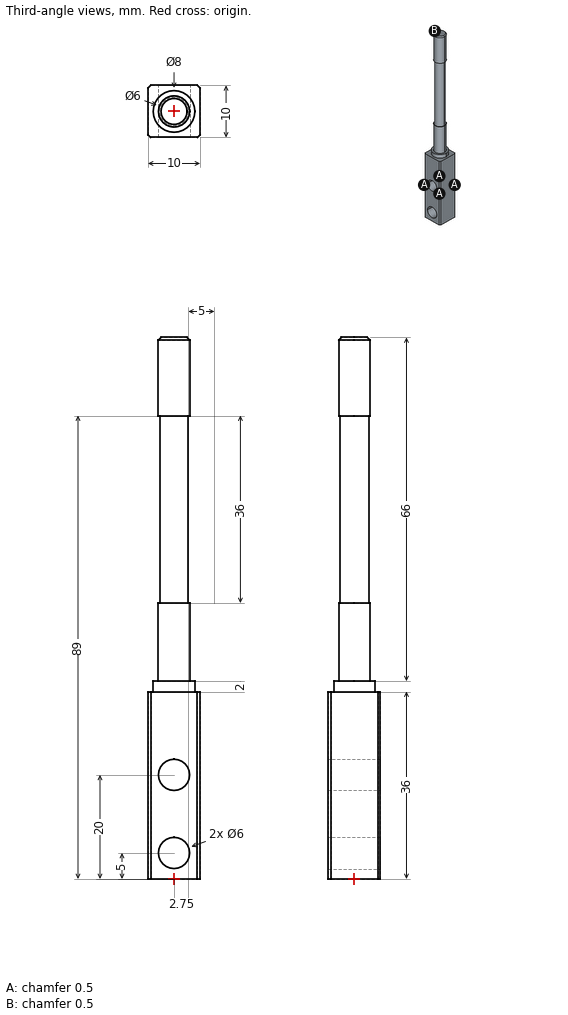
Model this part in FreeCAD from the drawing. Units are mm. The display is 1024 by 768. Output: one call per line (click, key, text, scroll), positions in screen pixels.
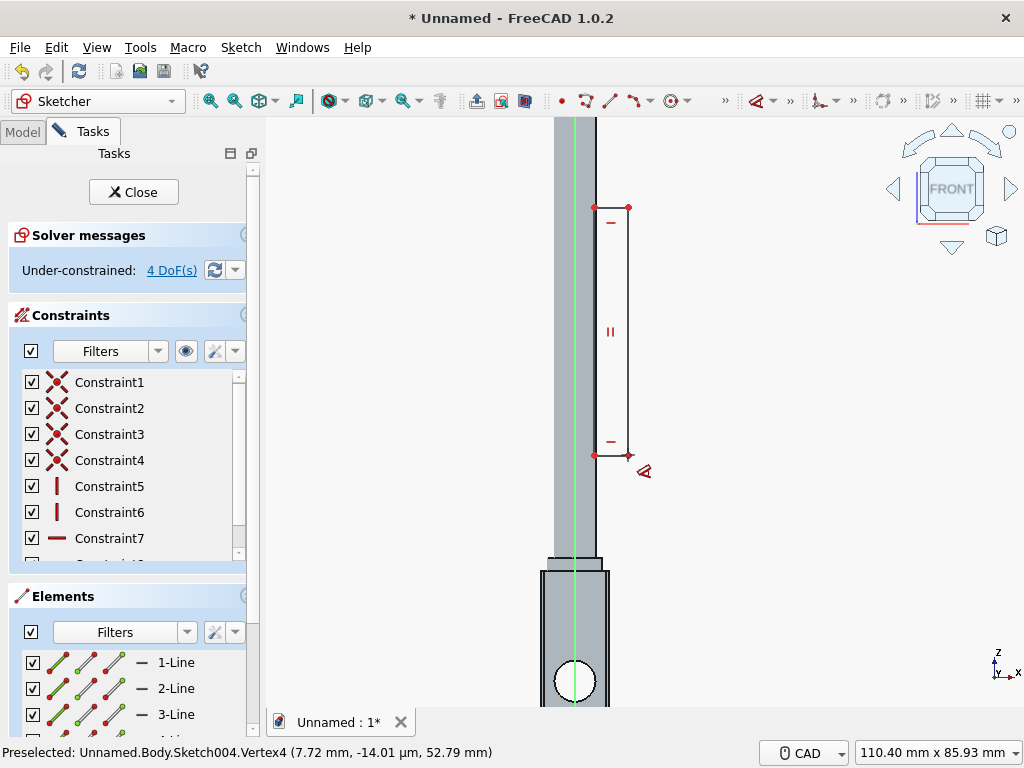
scroll(604, 456, up, 2)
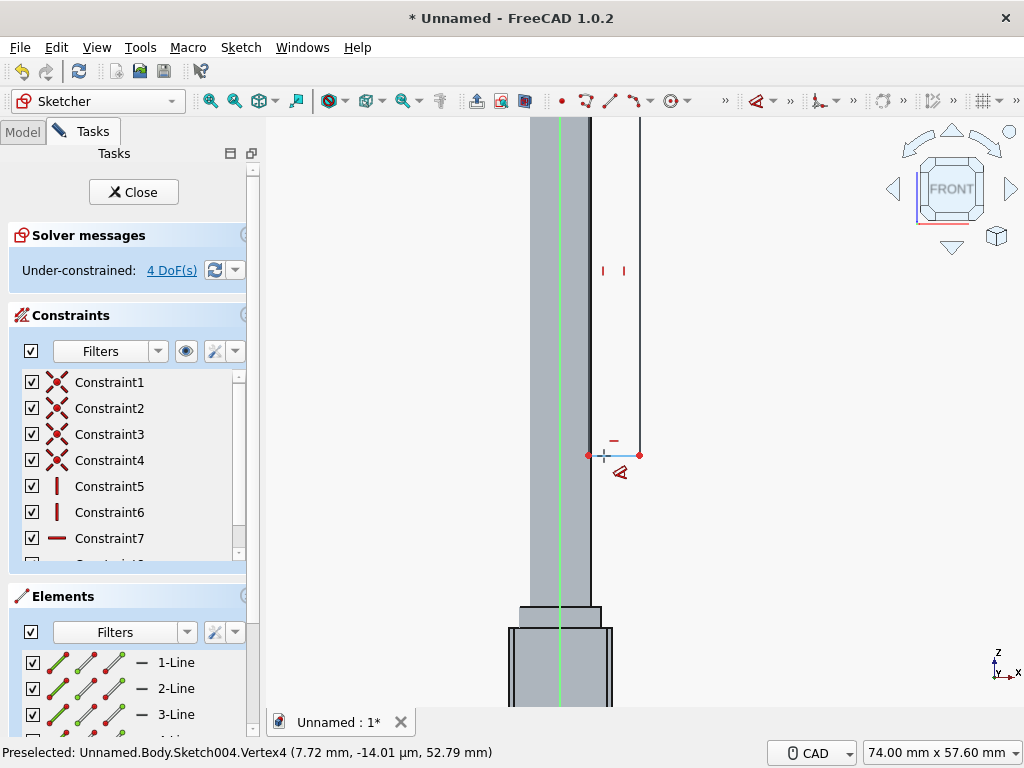
click(604, 456)
click(614, 422)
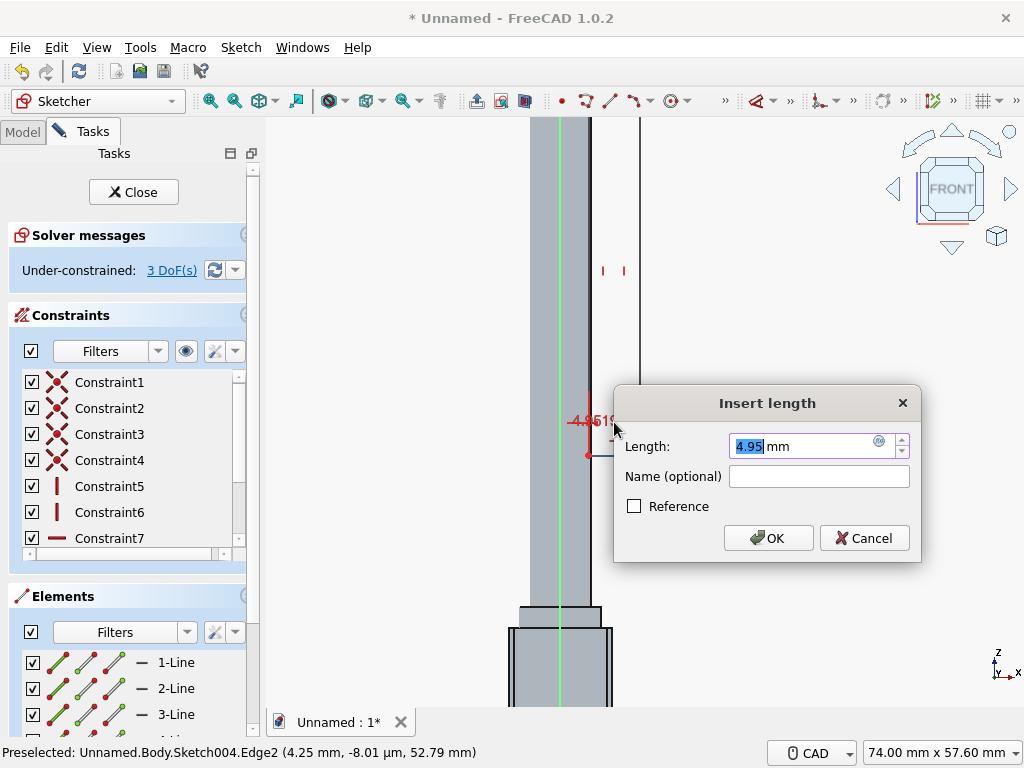
text(5)
key(Return)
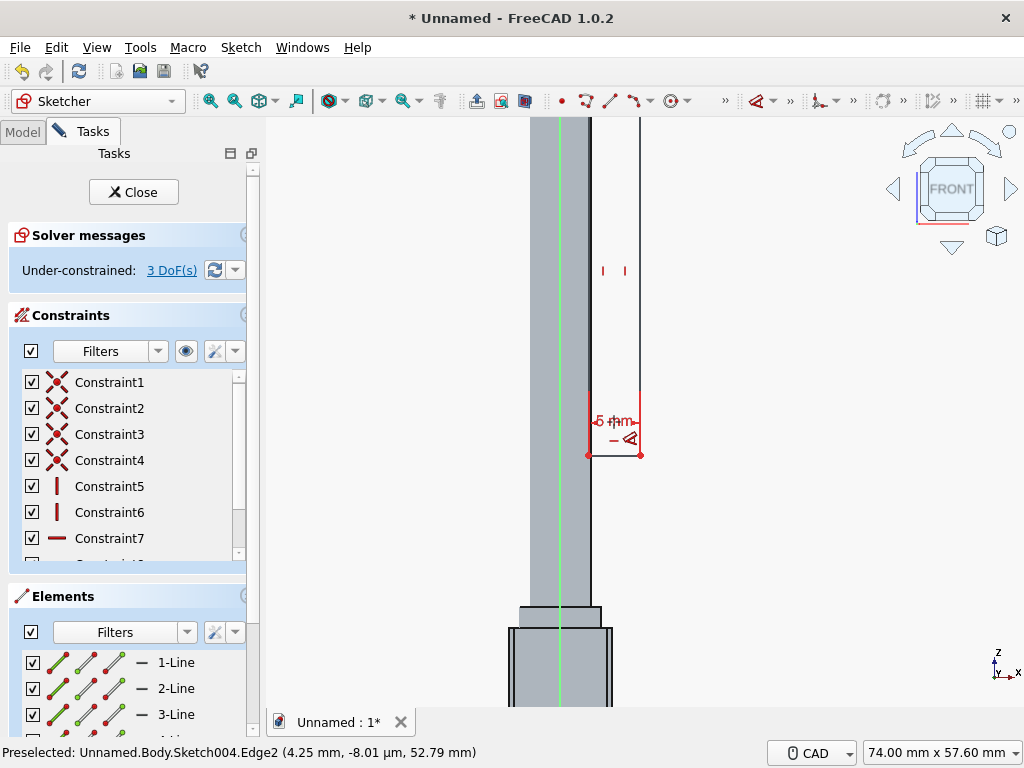
click(589, 197)
click(623, 300)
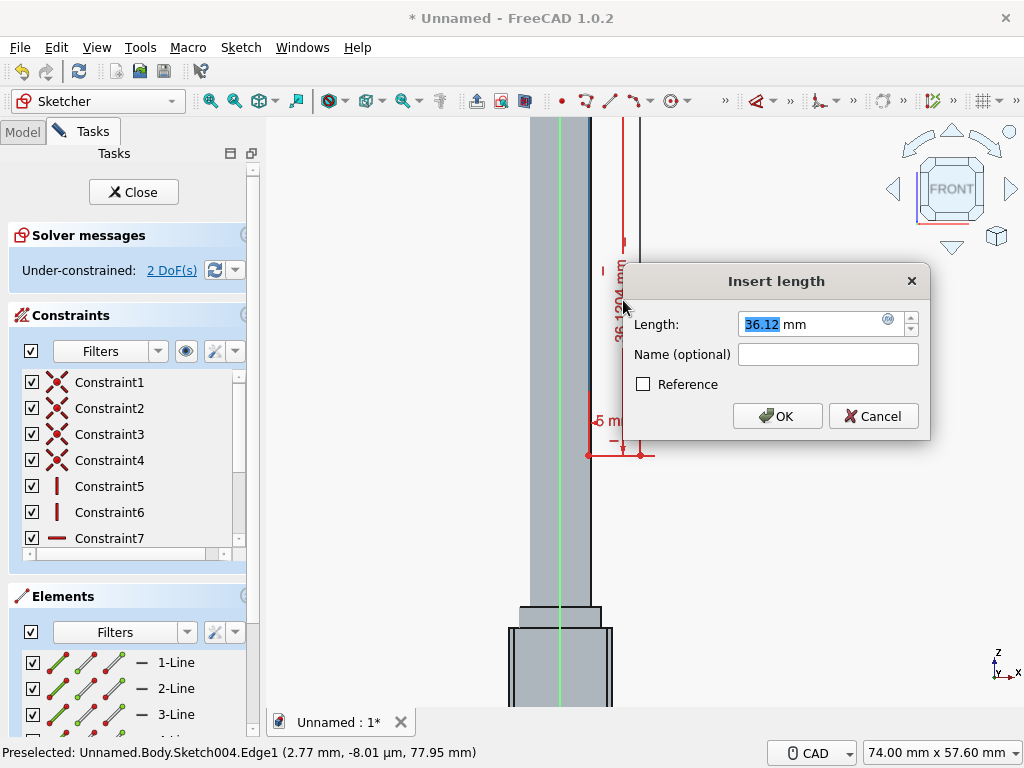
text(36)
key(Return)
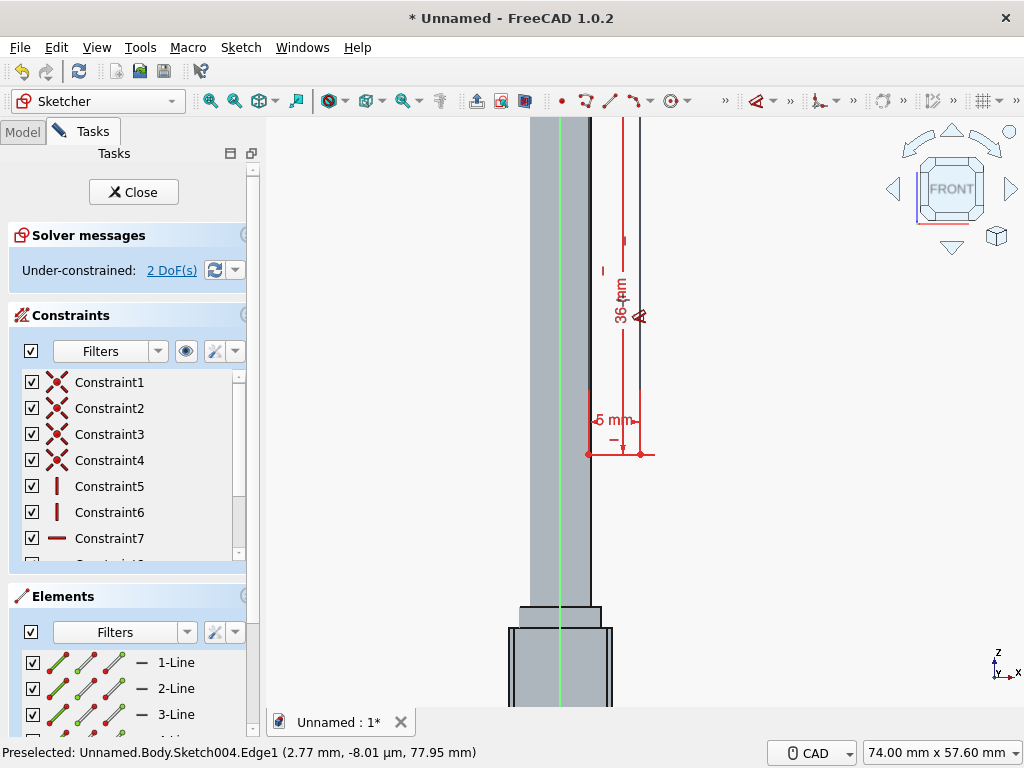
scroll(557, 307, down, 4)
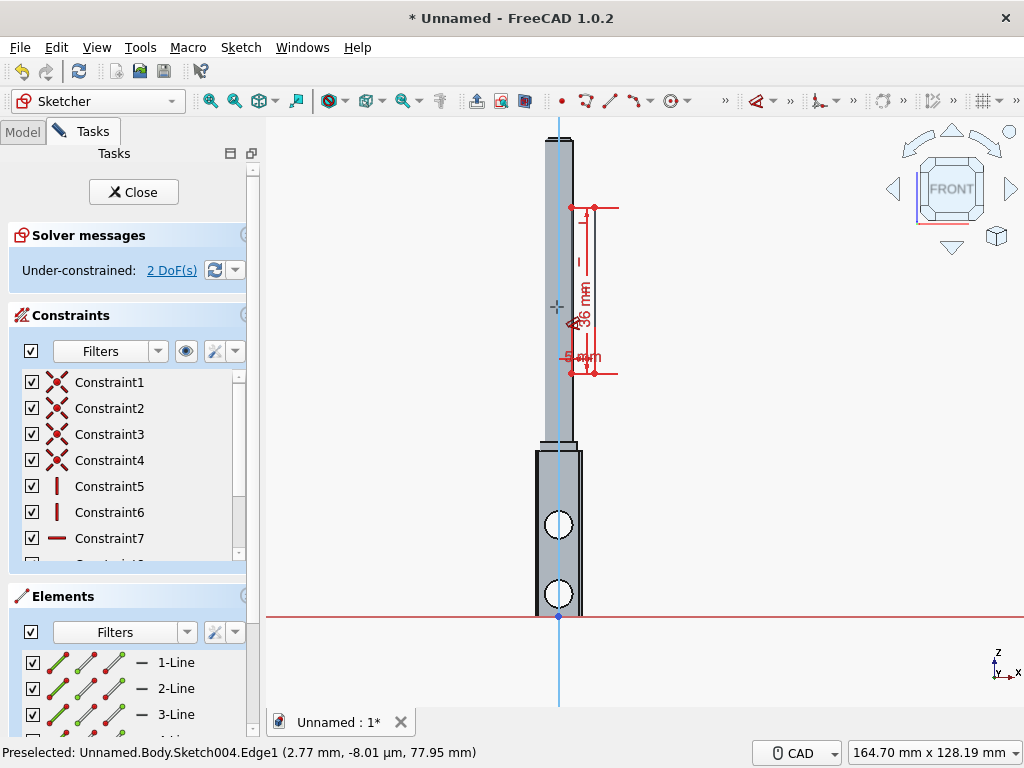
click(572, 208)
click(525, 412)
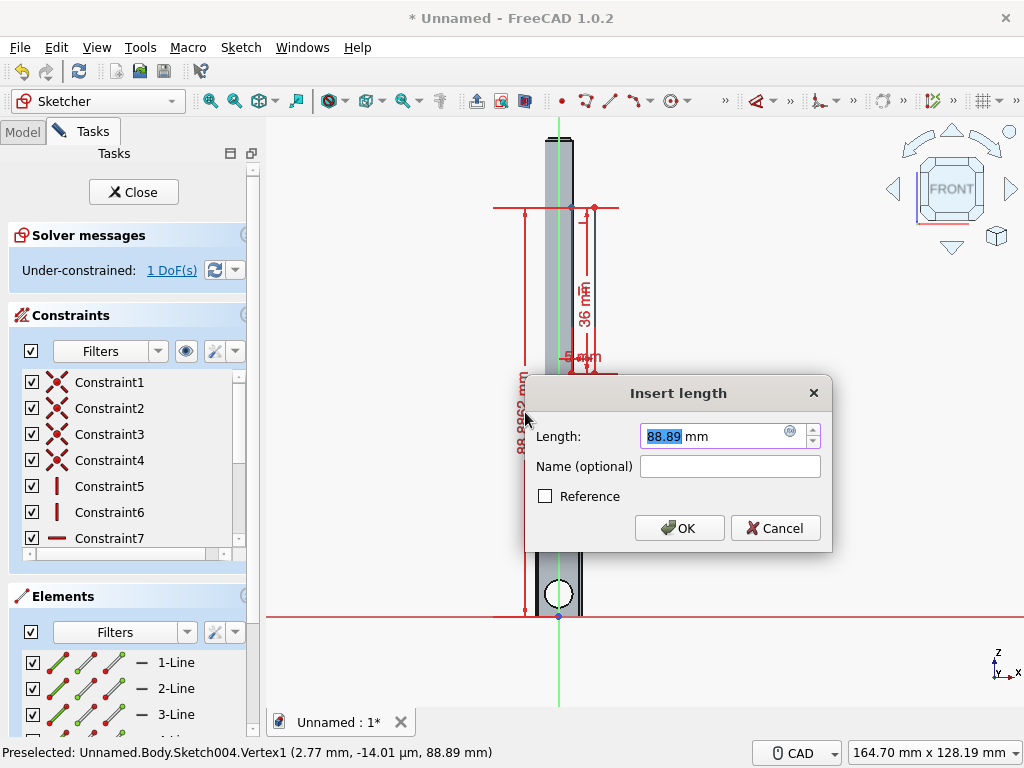
text(89)
key(Return)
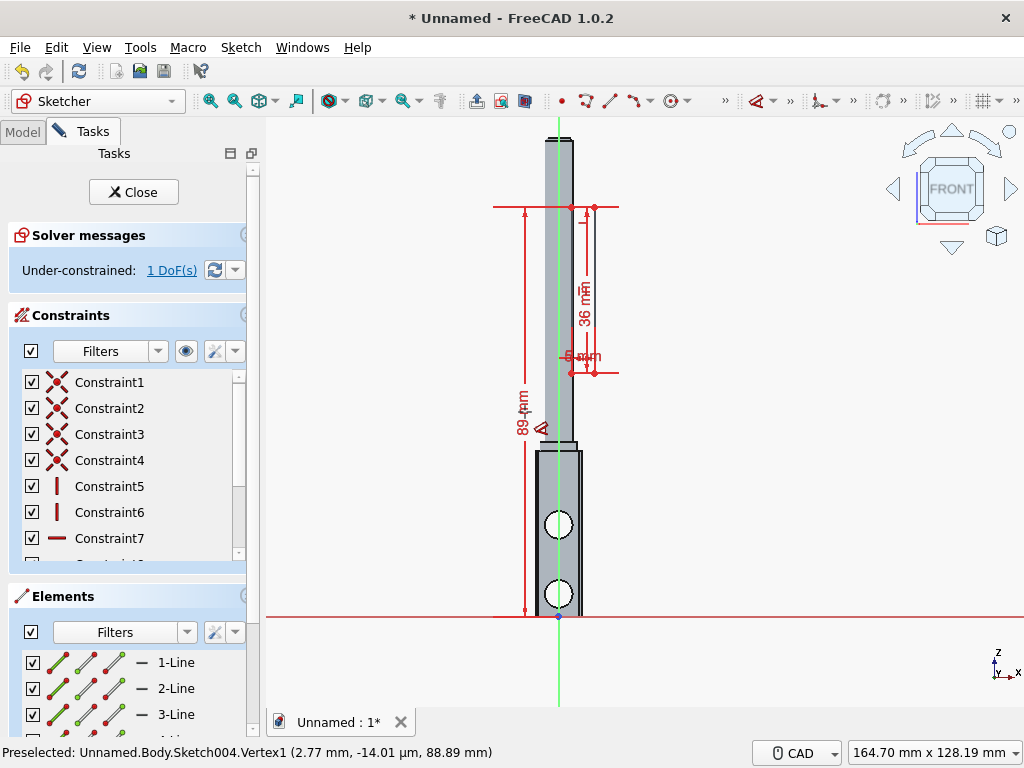
scroll(572, 207, up, 6)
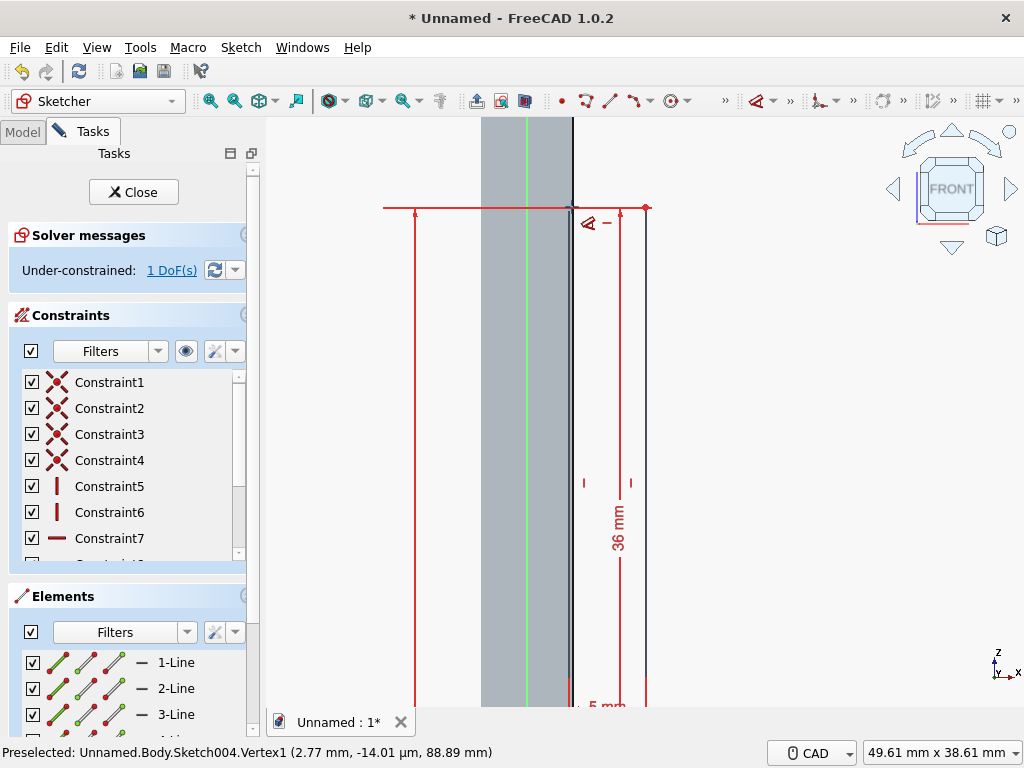
click(569, 208)
click(548, 174)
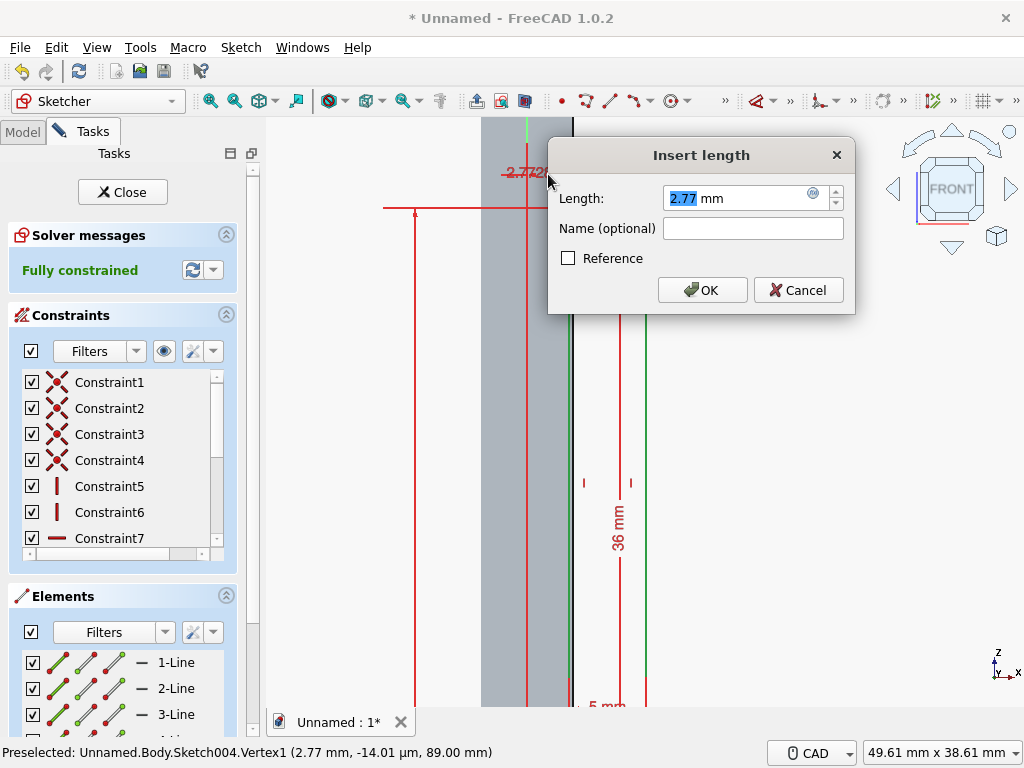
text(2.75)
key(Return)
key(Escape)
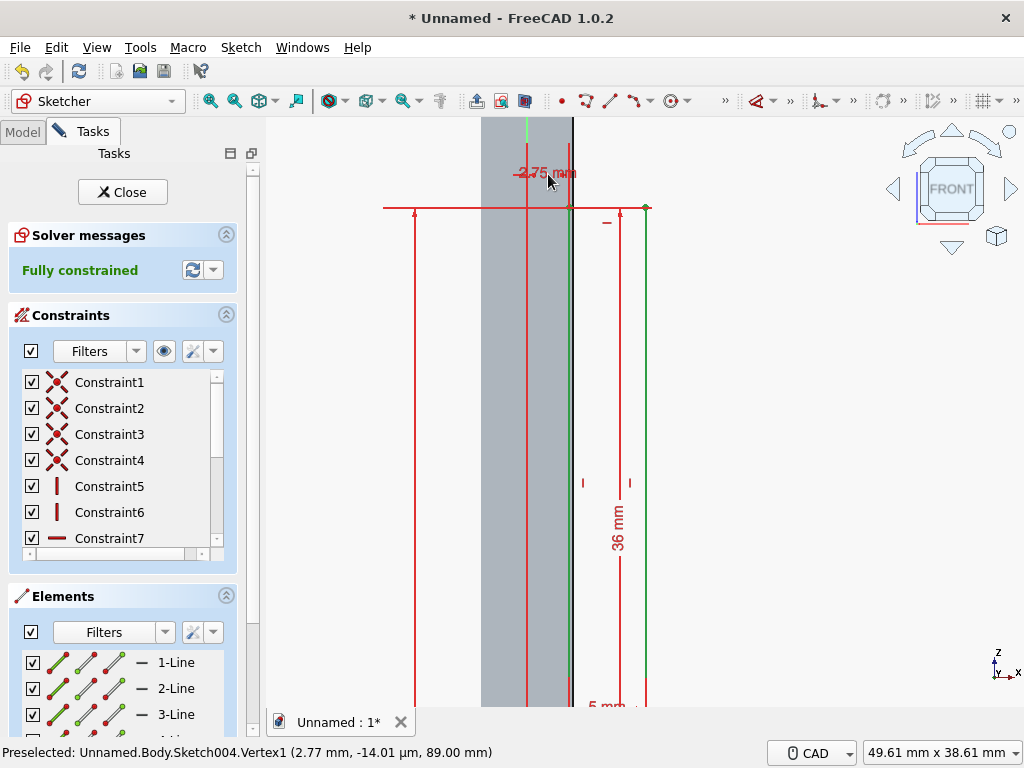
click(123, 192)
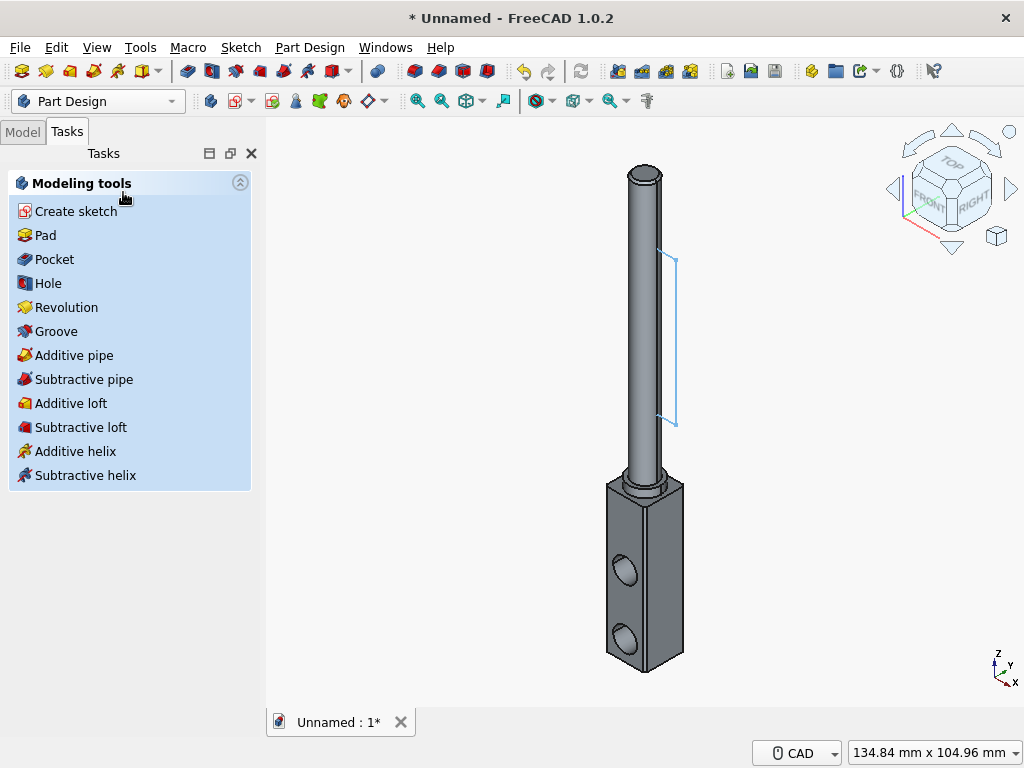
click(236, 72)